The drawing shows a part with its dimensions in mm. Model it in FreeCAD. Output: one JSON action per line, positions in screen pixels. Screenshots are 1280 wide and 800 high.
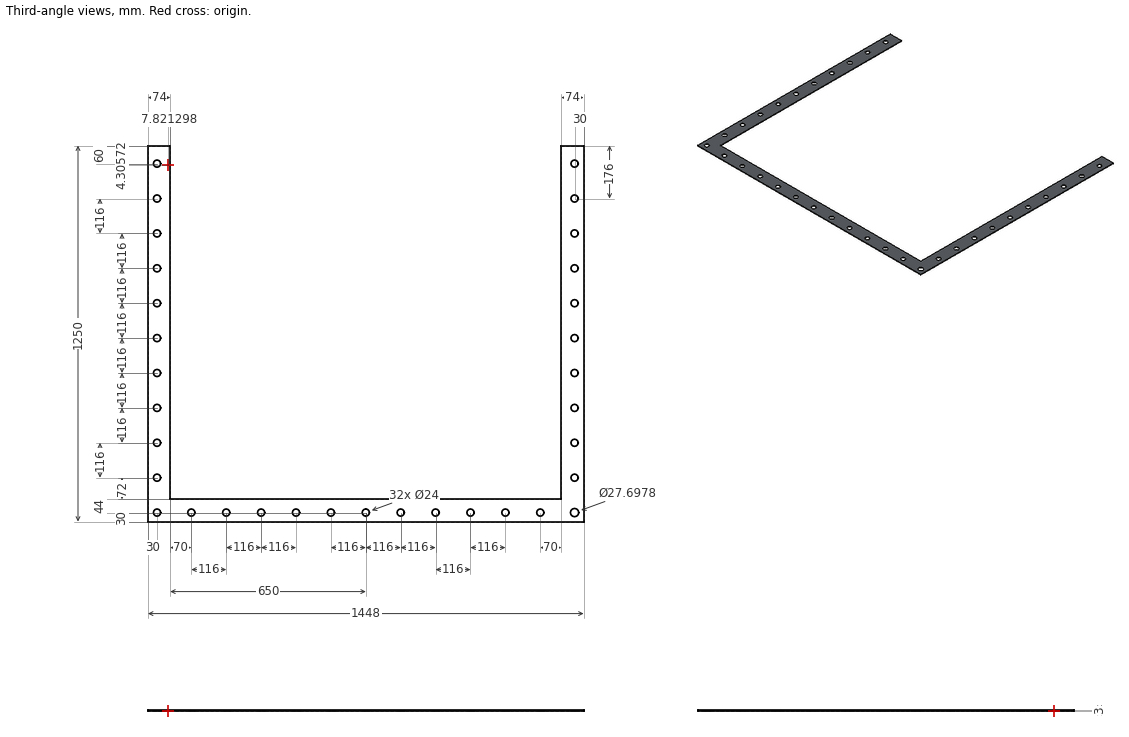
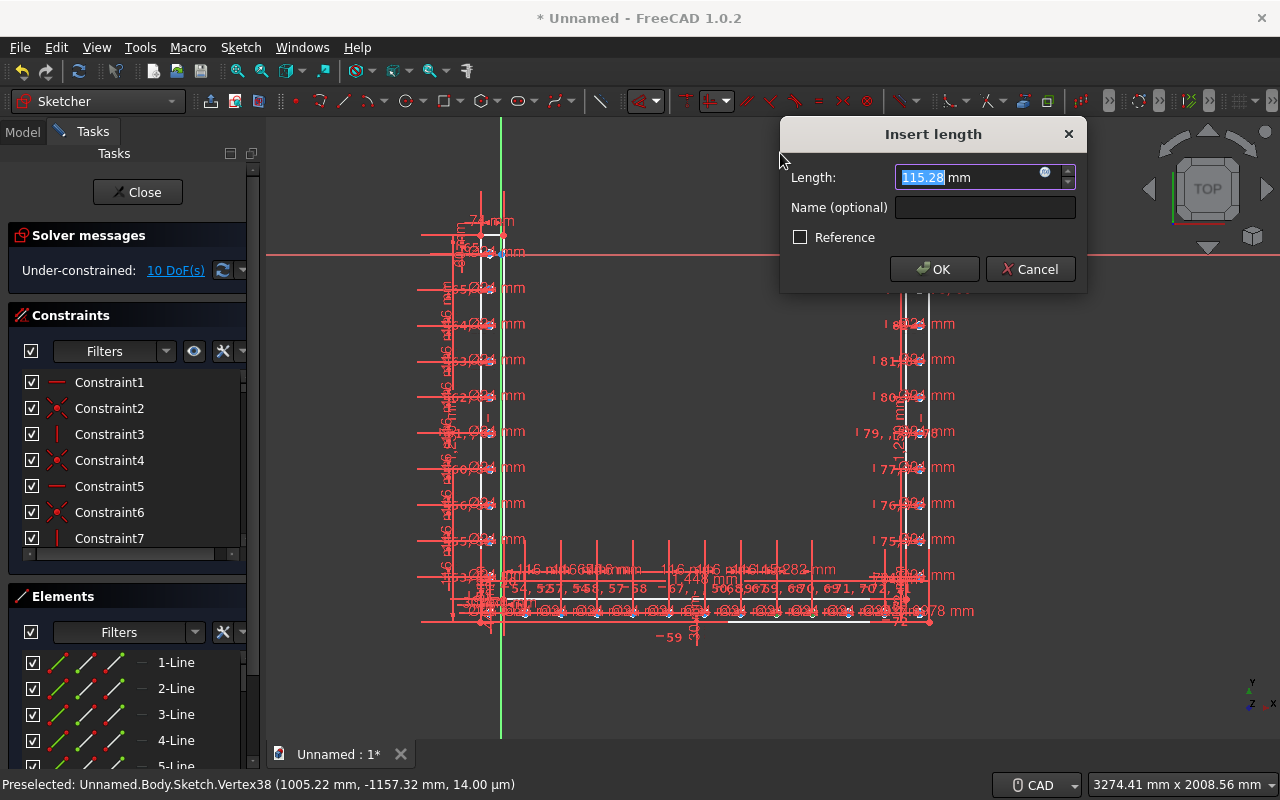
{"action": "type", "text": "116"}
{"action": "key", "text": "Return"}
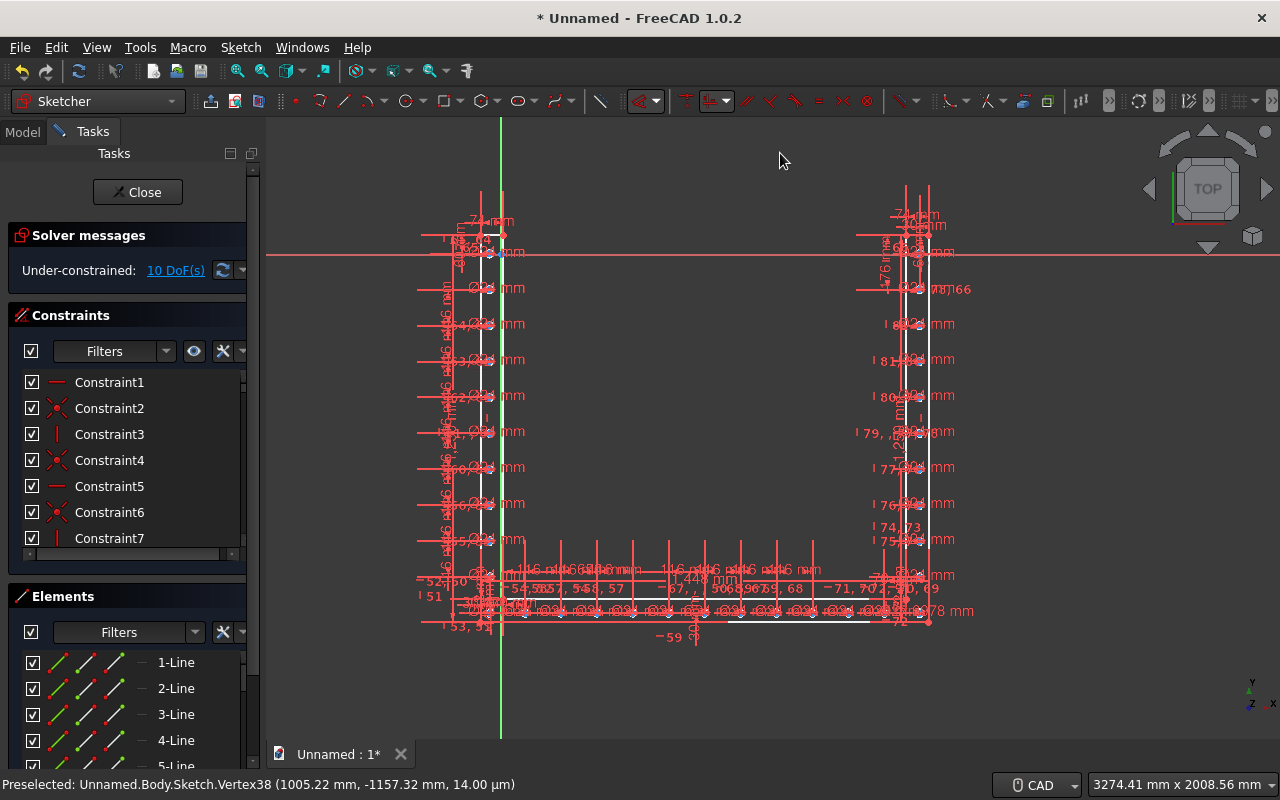
{"action": "left_click", "coordinate": [813, 613]}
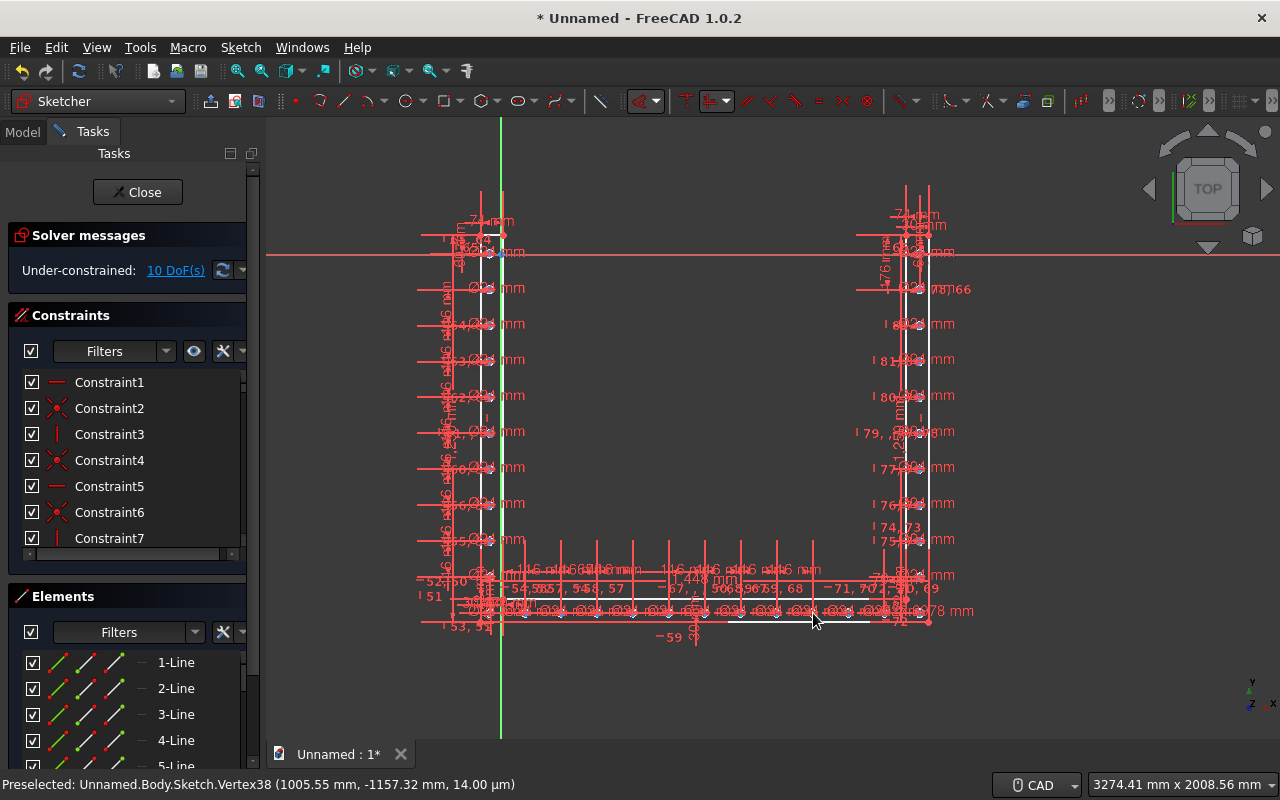
{"action": "left_click", "coordinate": [849, 613]}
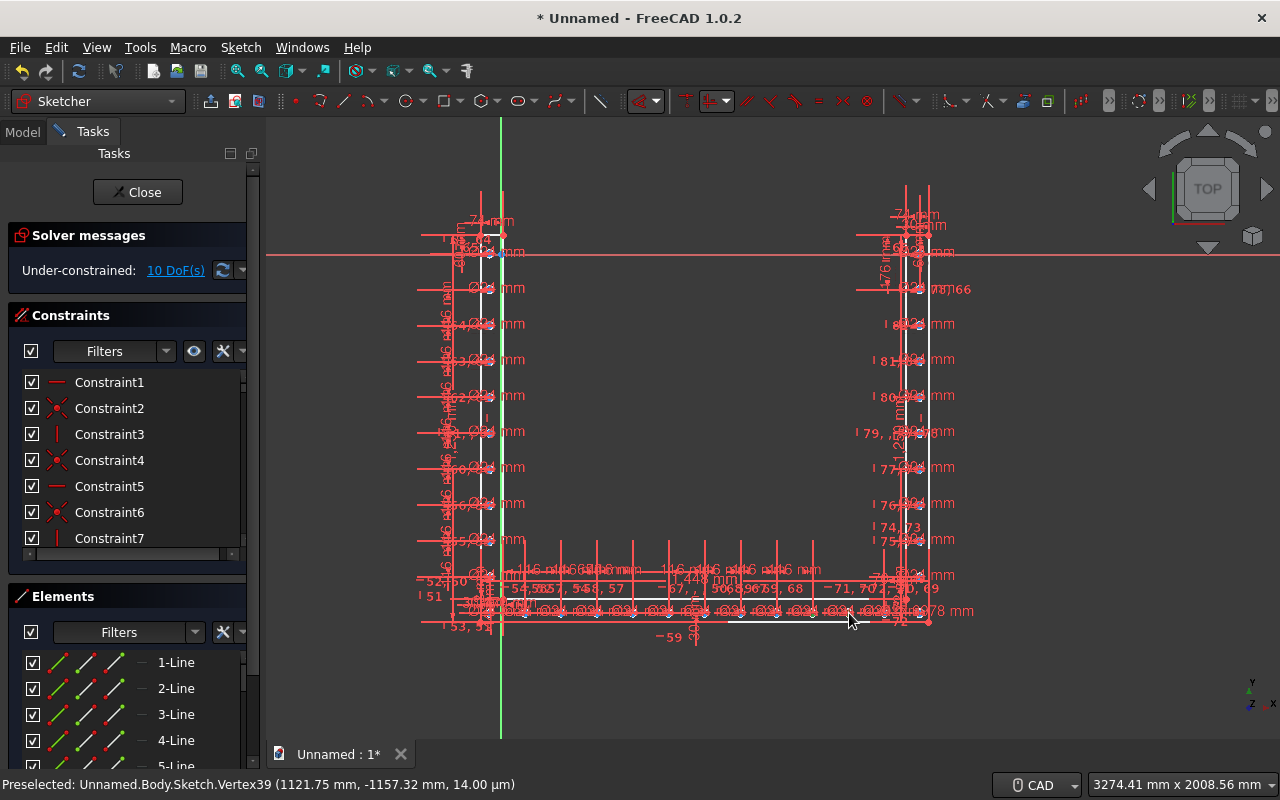
{"action": "left_click", "coordinate": [658, 102]}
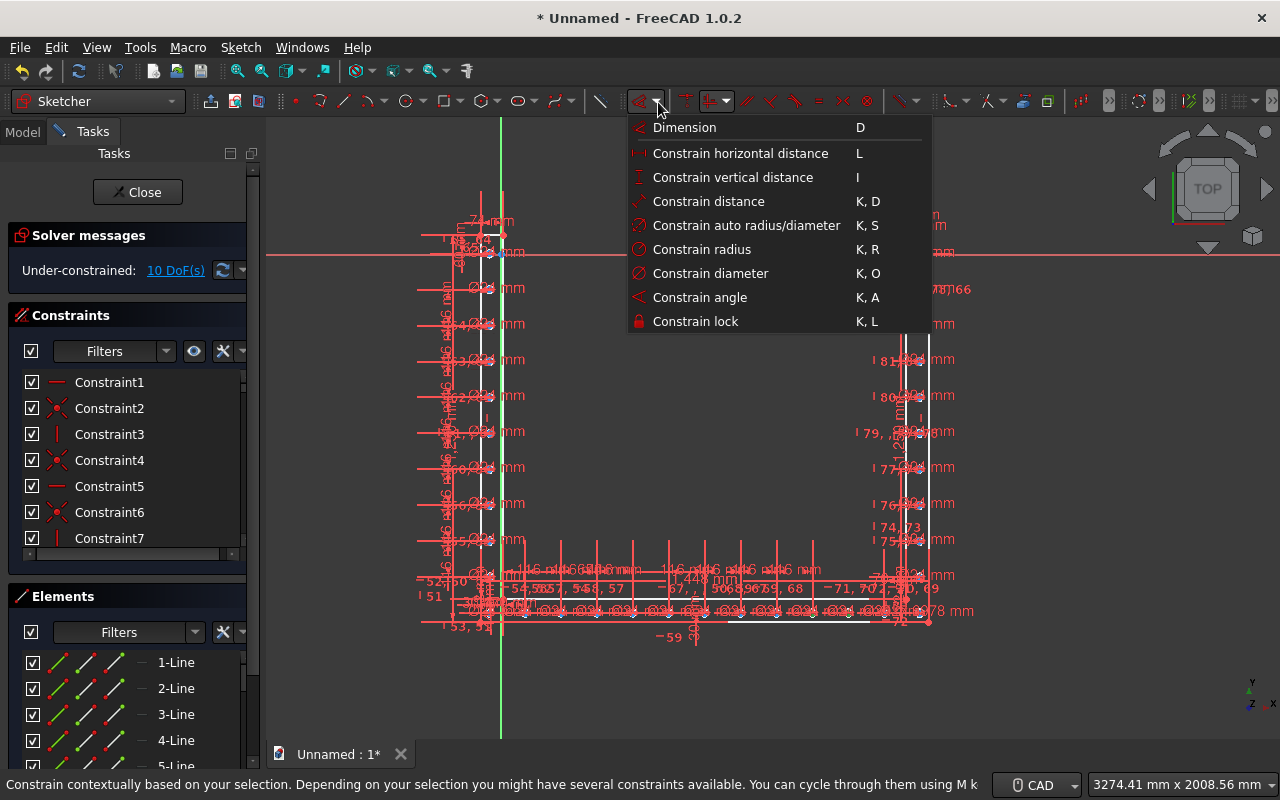
{"action": "left_click", "coordinate": [780, 153]}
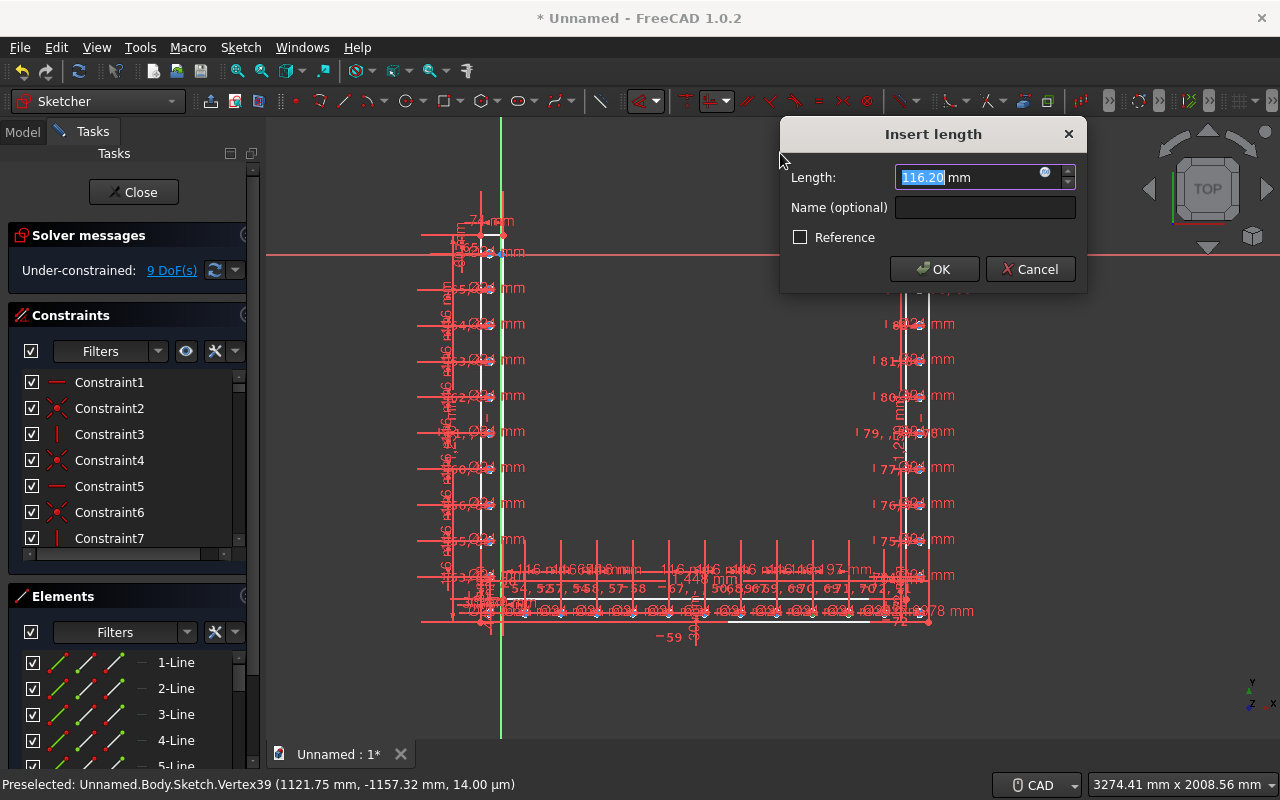
{"action": "type", "text": "116"}
{"action": "key", "text": "Return"}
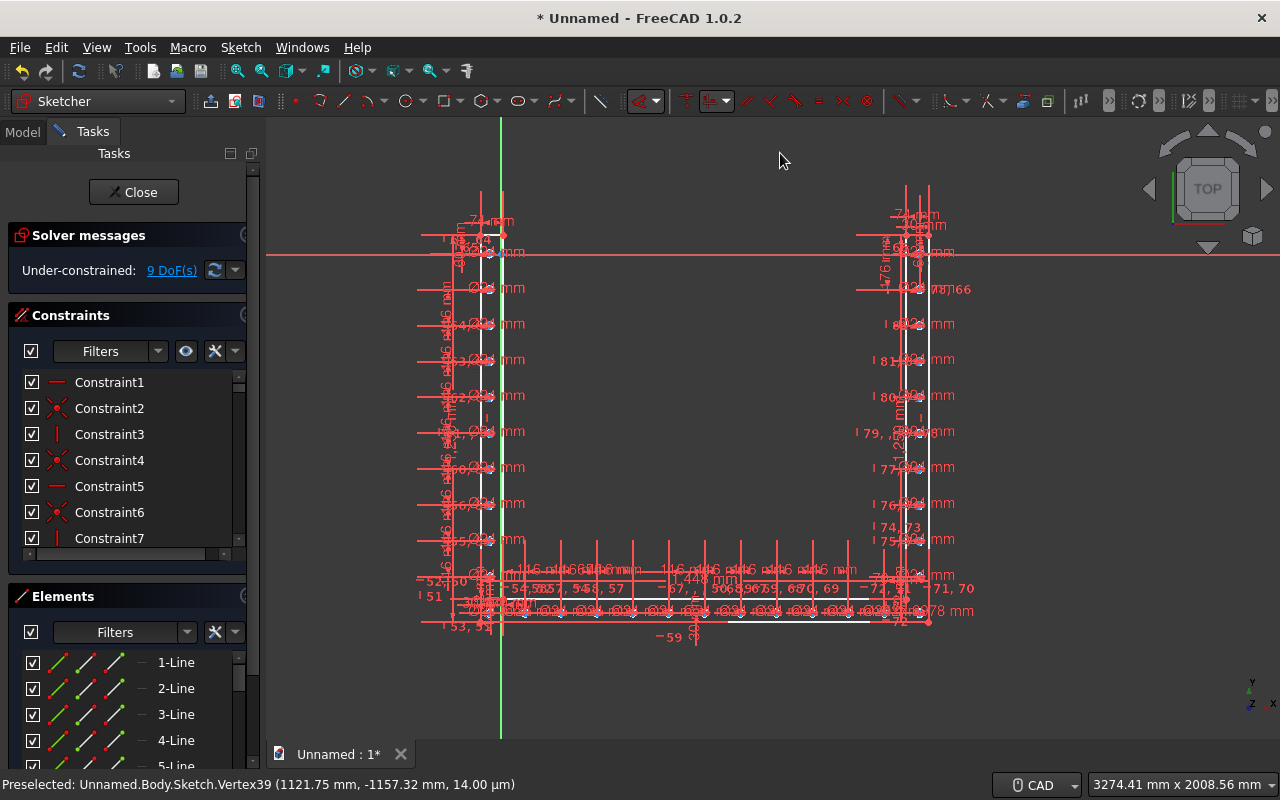
{"action": "left_click", "coordinate": [920, 577]}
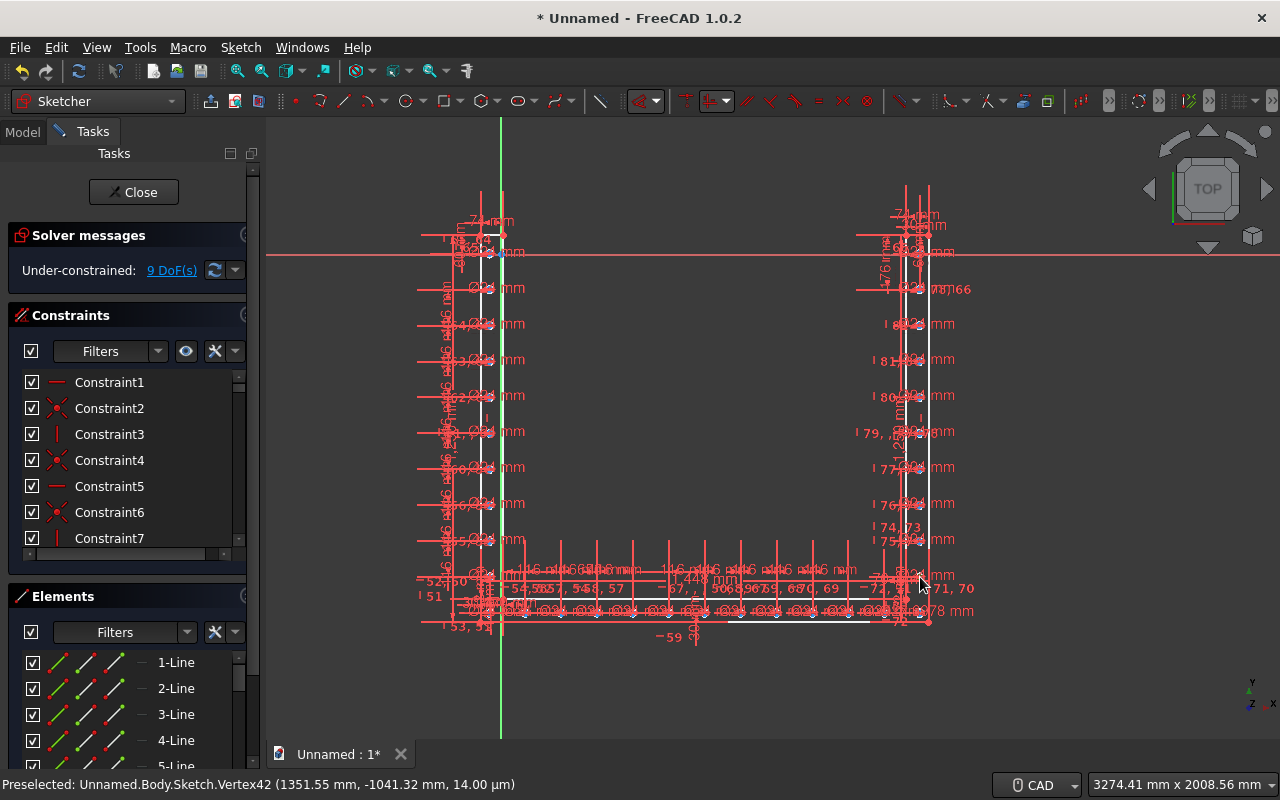
{"action": "left_click", "coordinate": [920, 541]}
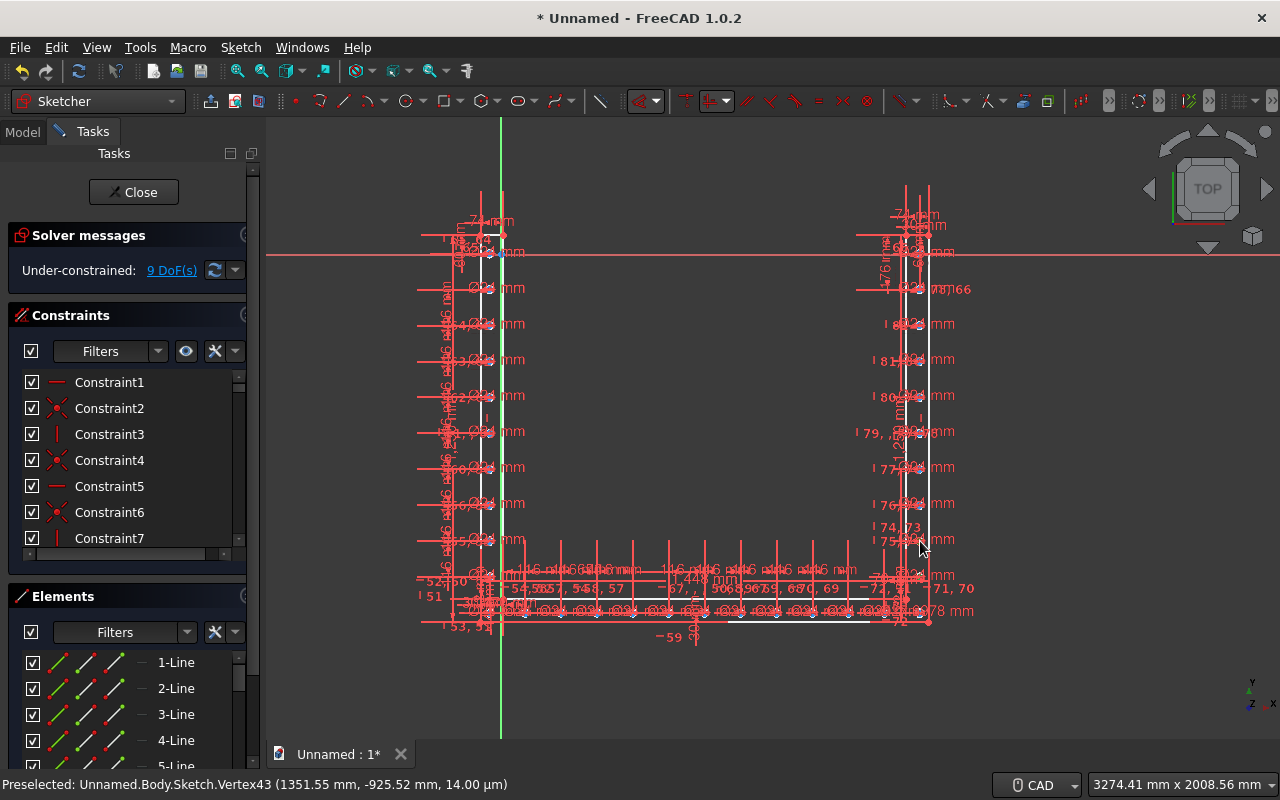
{"action": "key", "text": "i"}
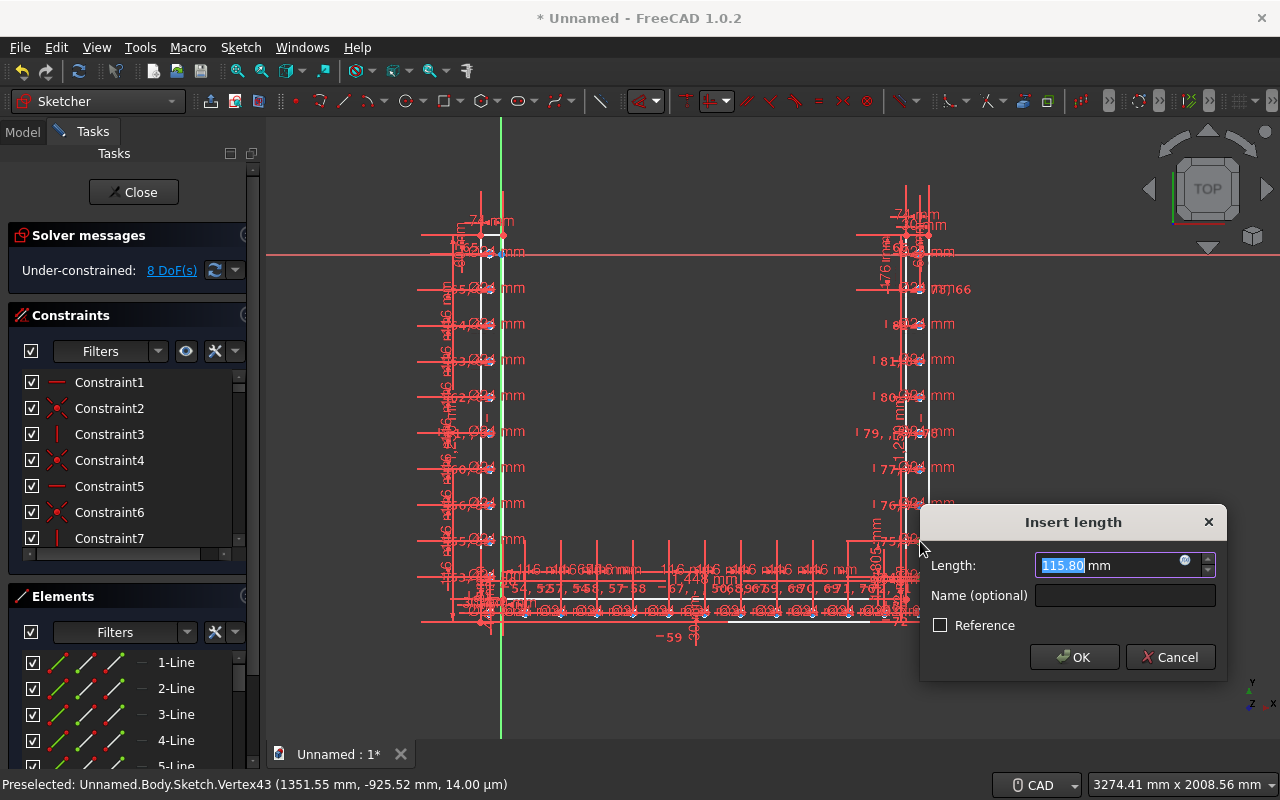
{"action": "type", "text": "116"}
{"action": "key", "text": "Return"}